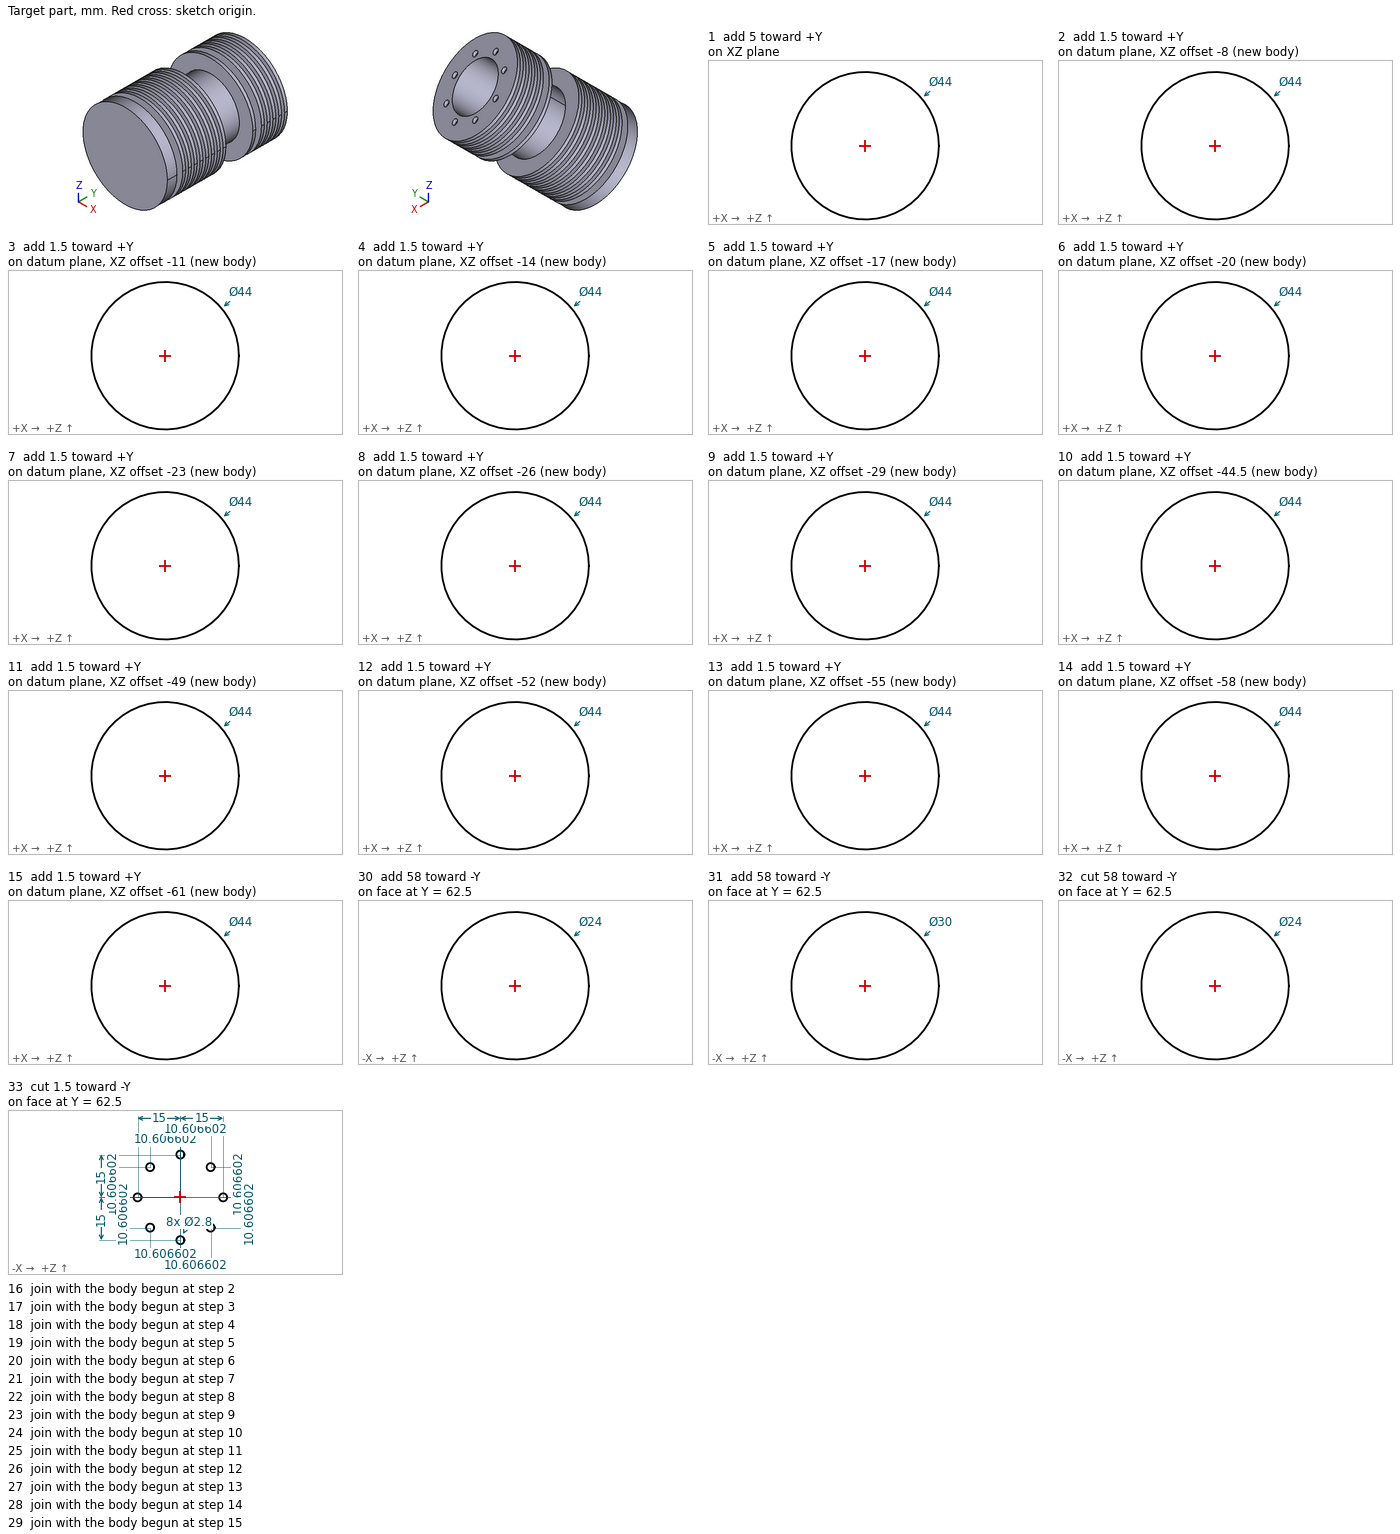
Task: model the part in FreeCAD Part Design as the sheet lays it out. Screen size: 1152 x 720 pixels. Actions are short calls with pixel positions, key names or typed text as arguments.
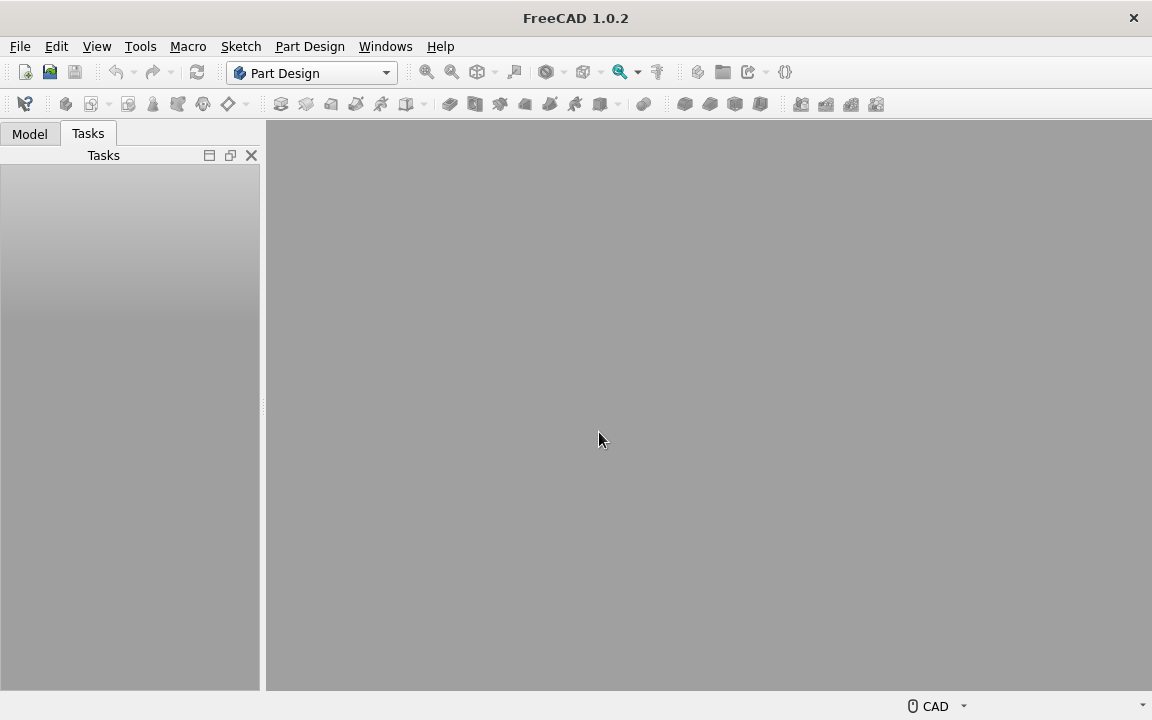
key(ctrl+n)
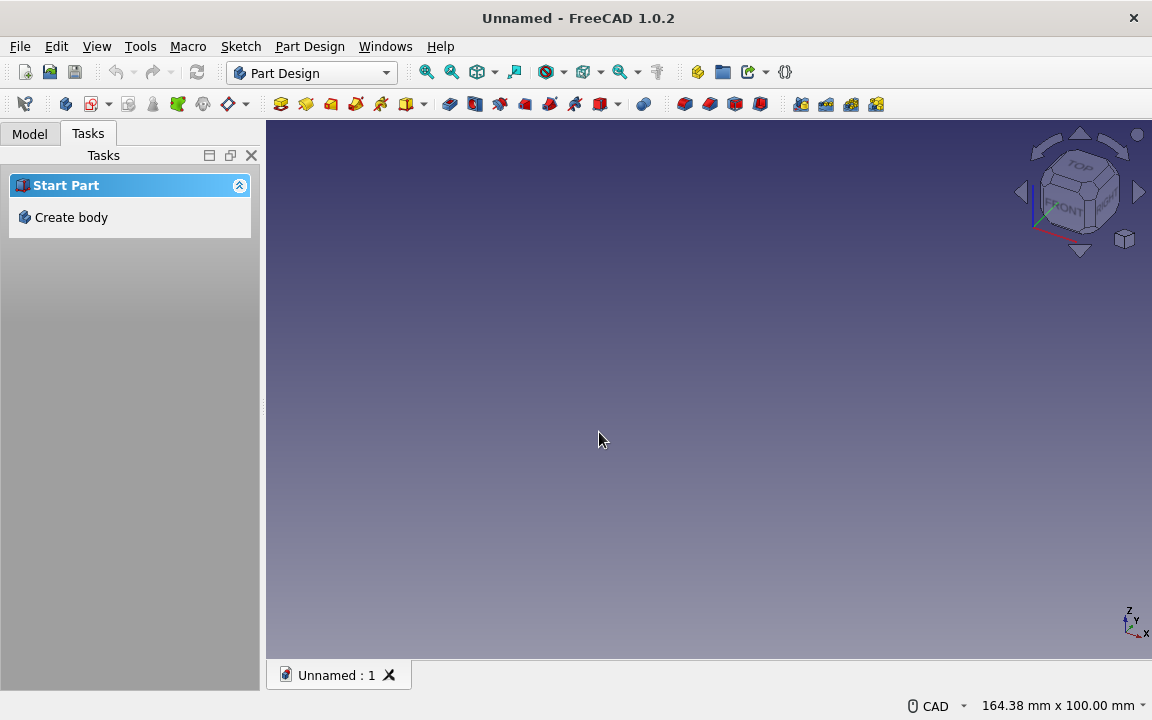
click(90, 104)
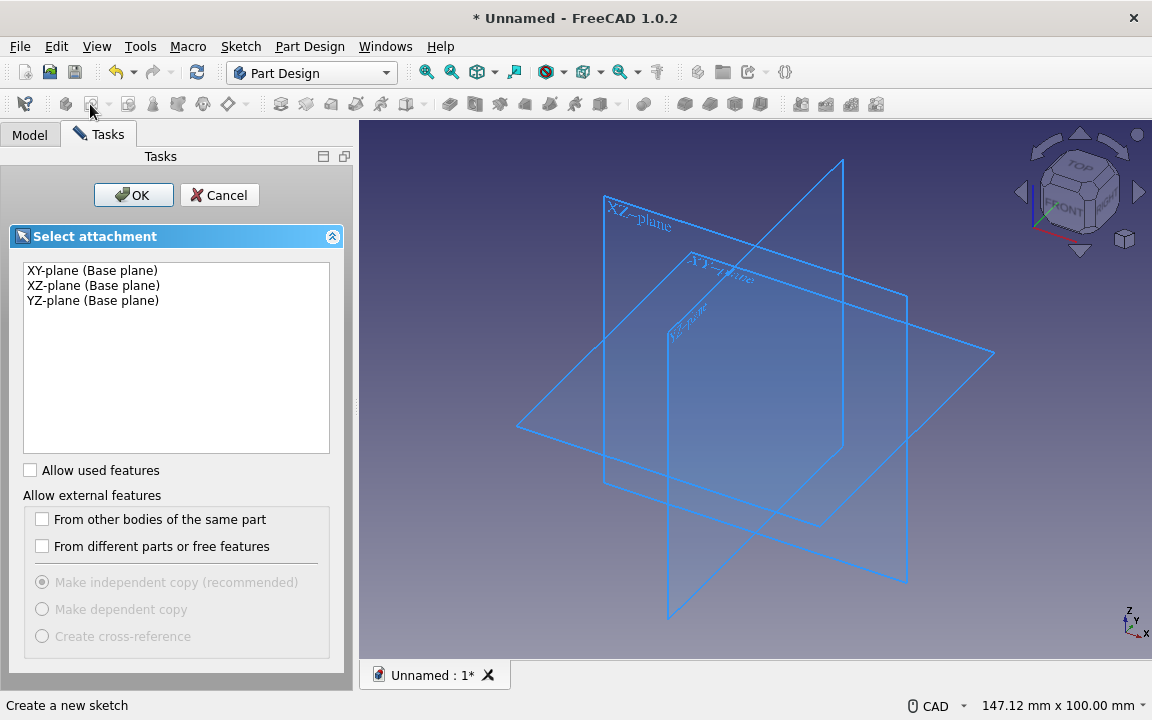
click(84, 286)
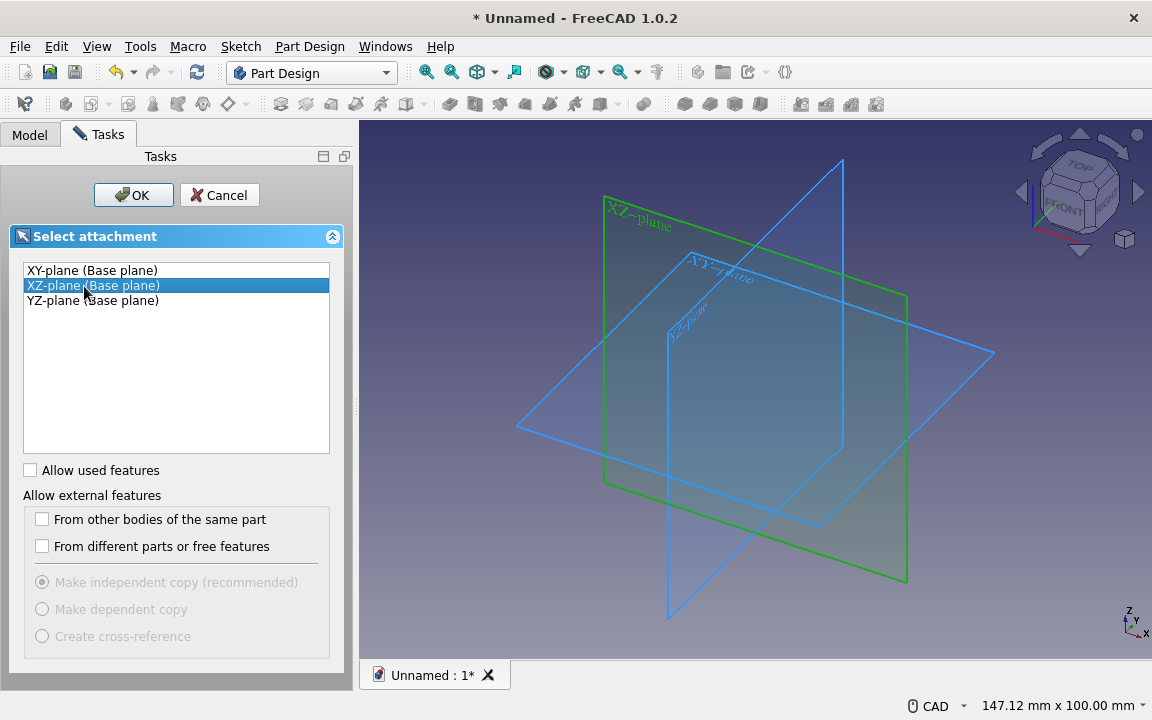
click(134, 195)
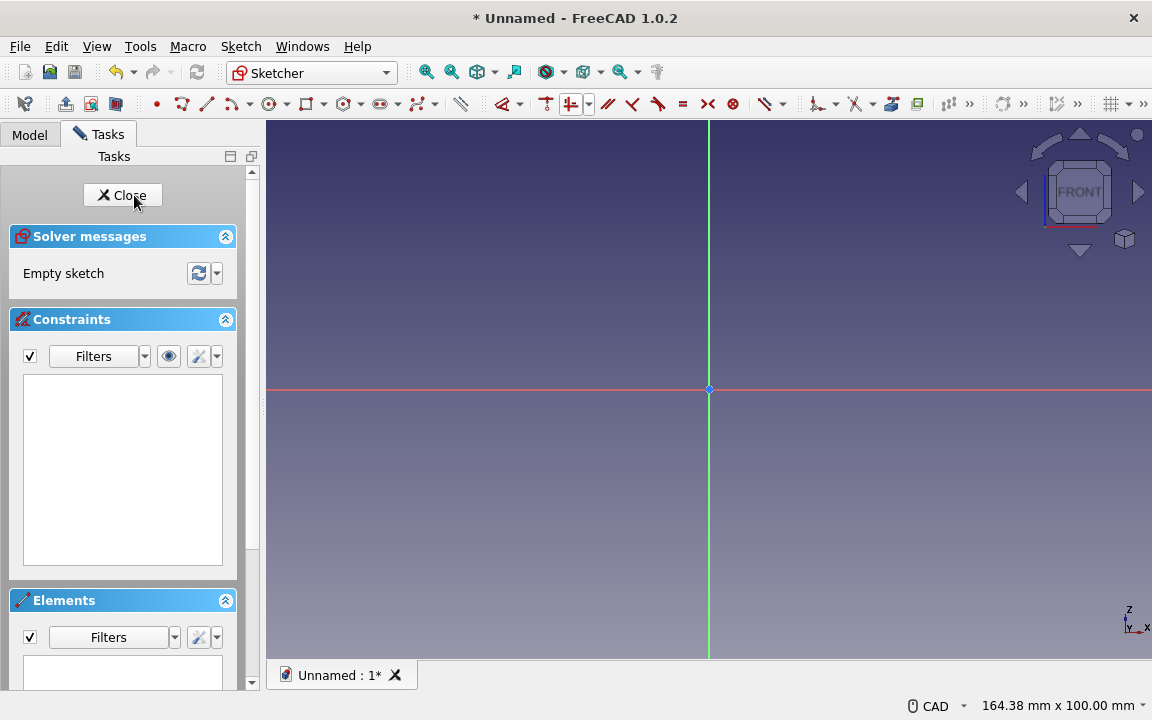
scroll(848, 390, up, 2)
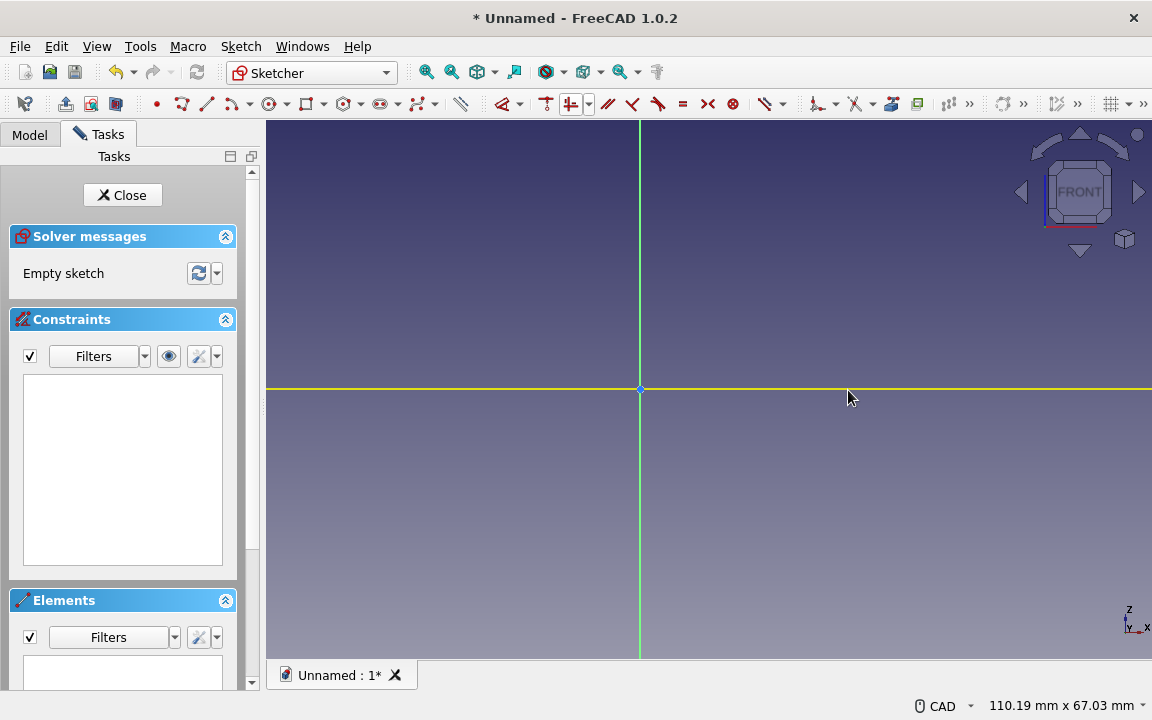
click(268, 104)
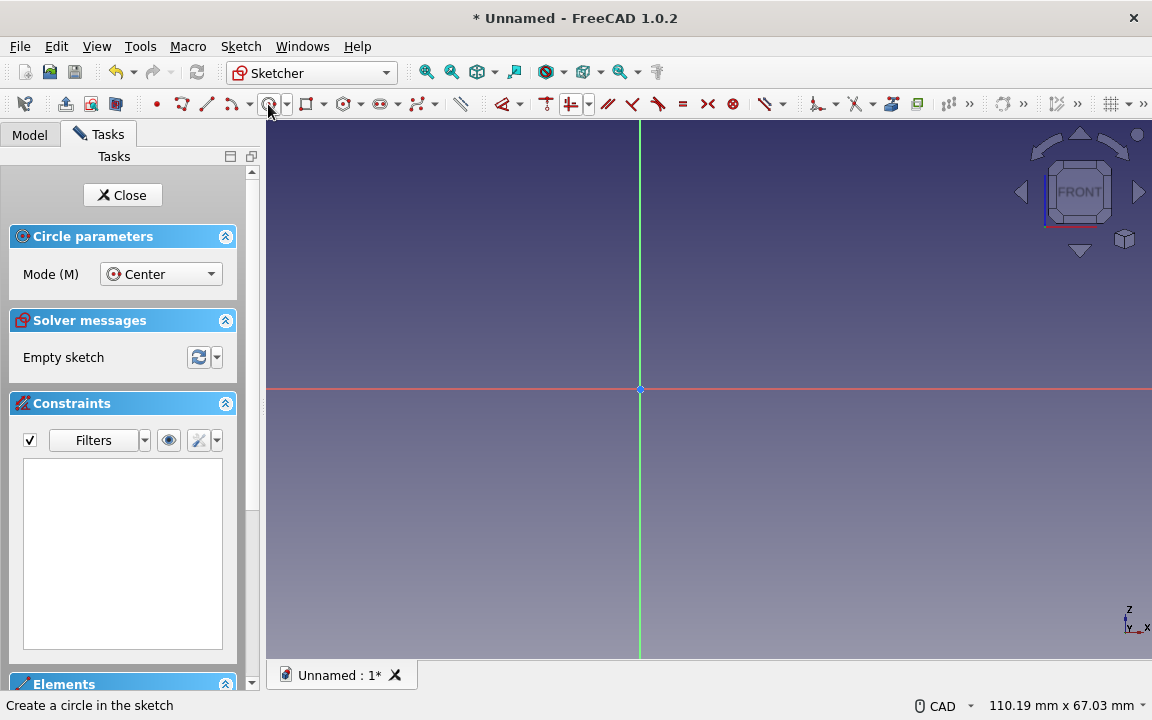
click(640, 389)
click(765, 264)
key(Escape)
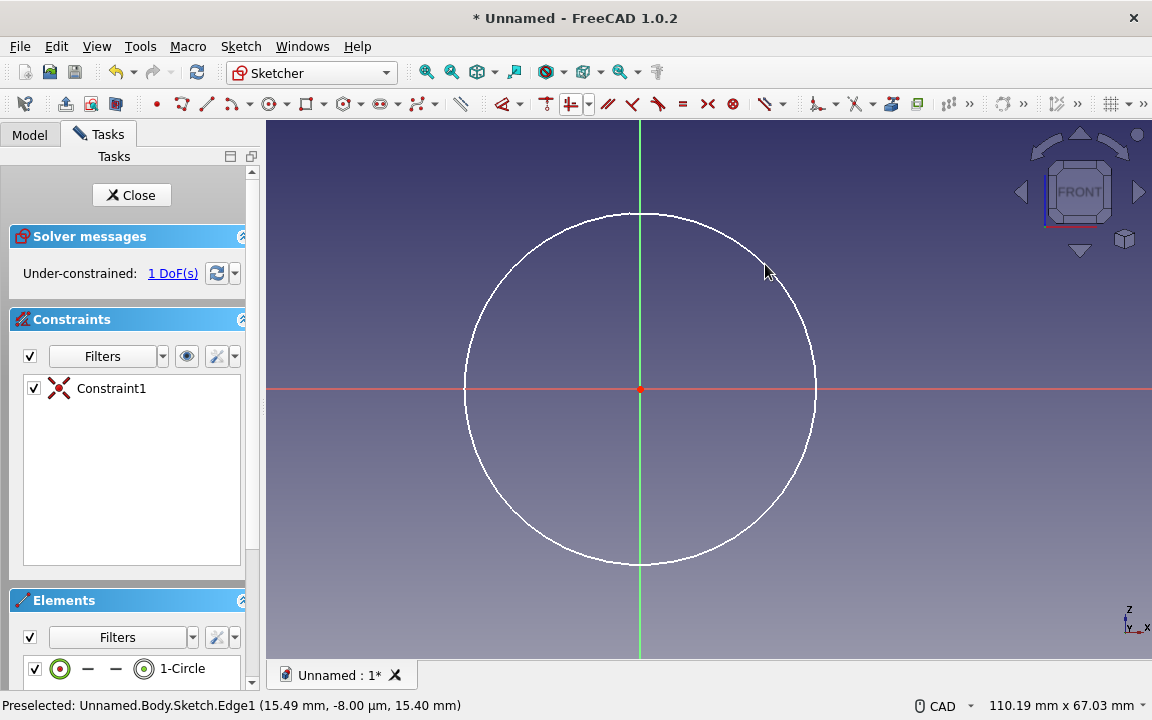
click(764, 264)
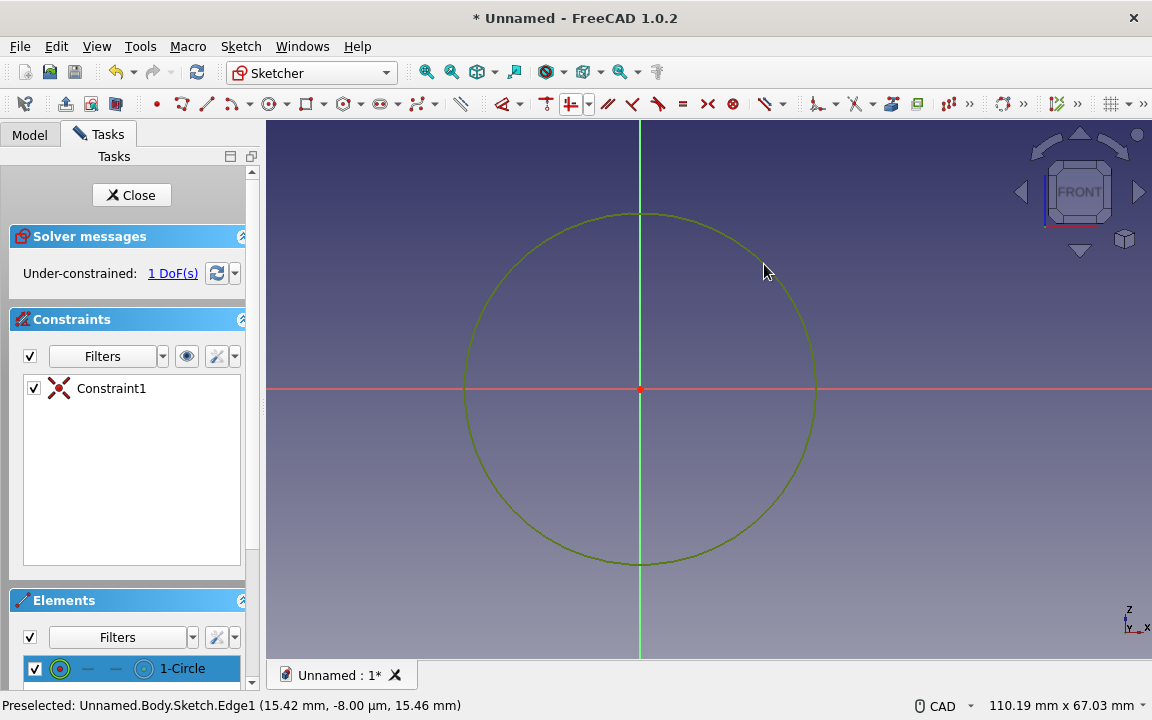
key(k)
key(o)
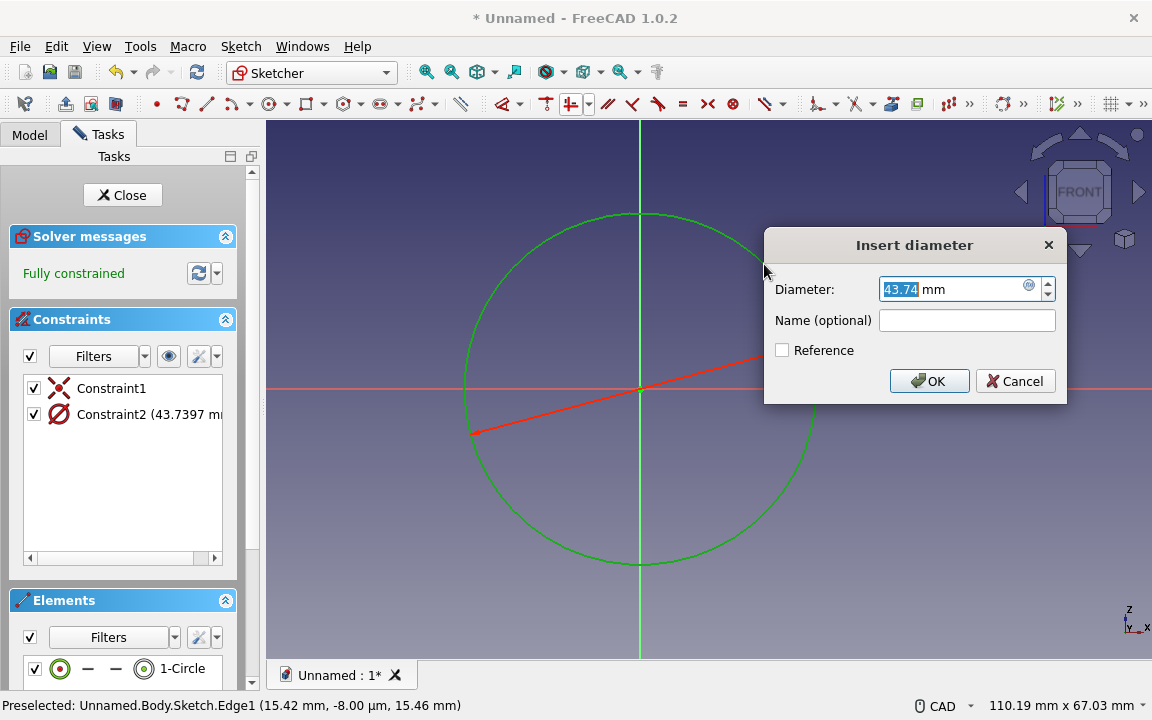
text(44)
key(Return)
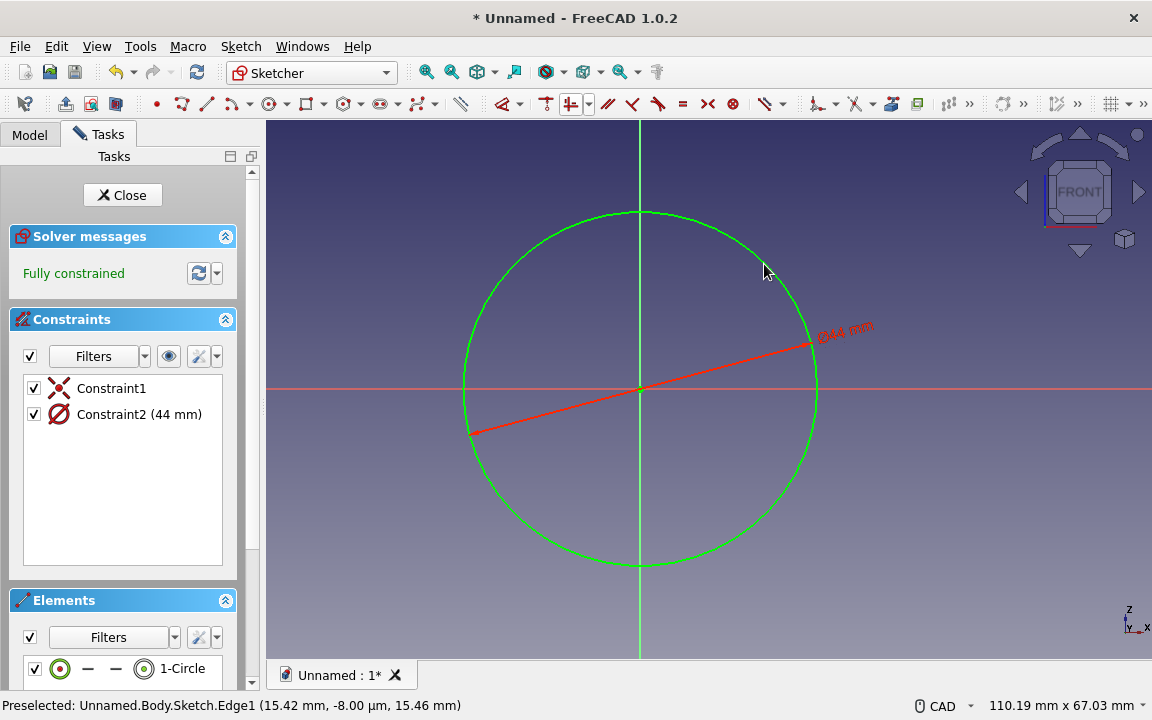
click(123, 195)